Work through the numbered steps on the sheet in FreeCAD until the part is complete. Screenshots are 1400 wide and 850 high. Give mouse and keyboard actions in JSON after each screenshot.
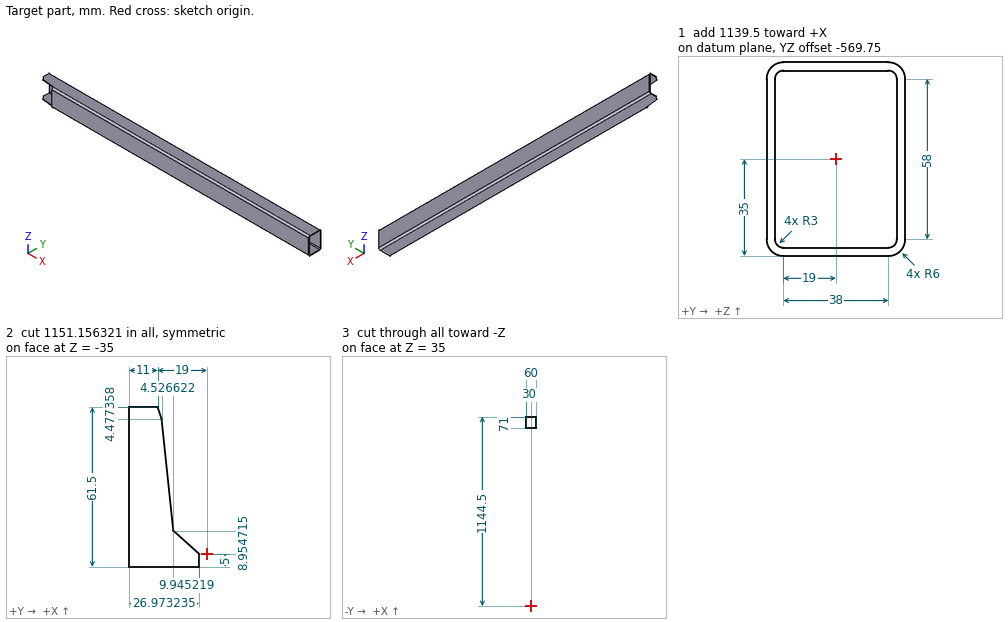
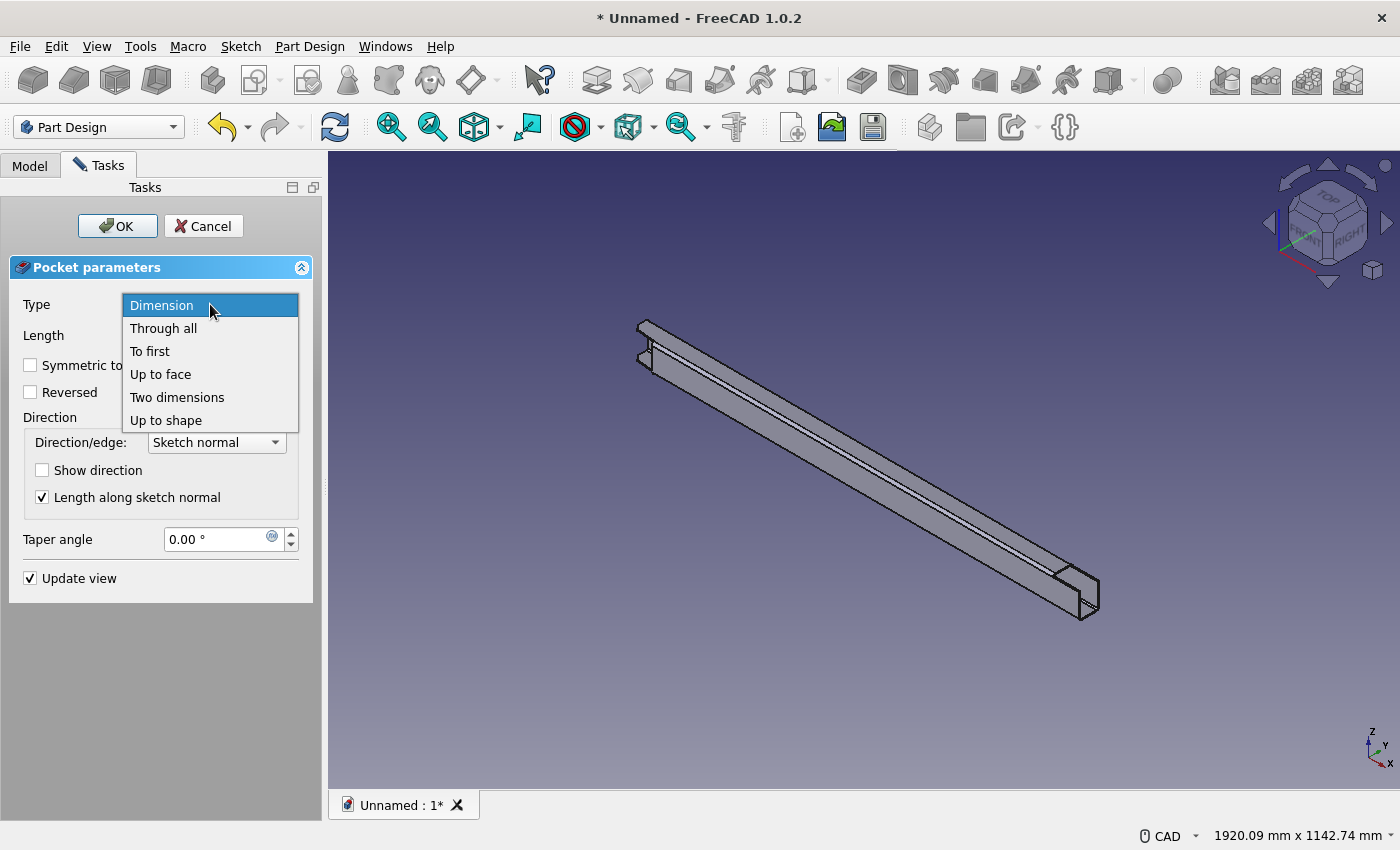
{"action": "left_click", "coordinate": [208, 328]}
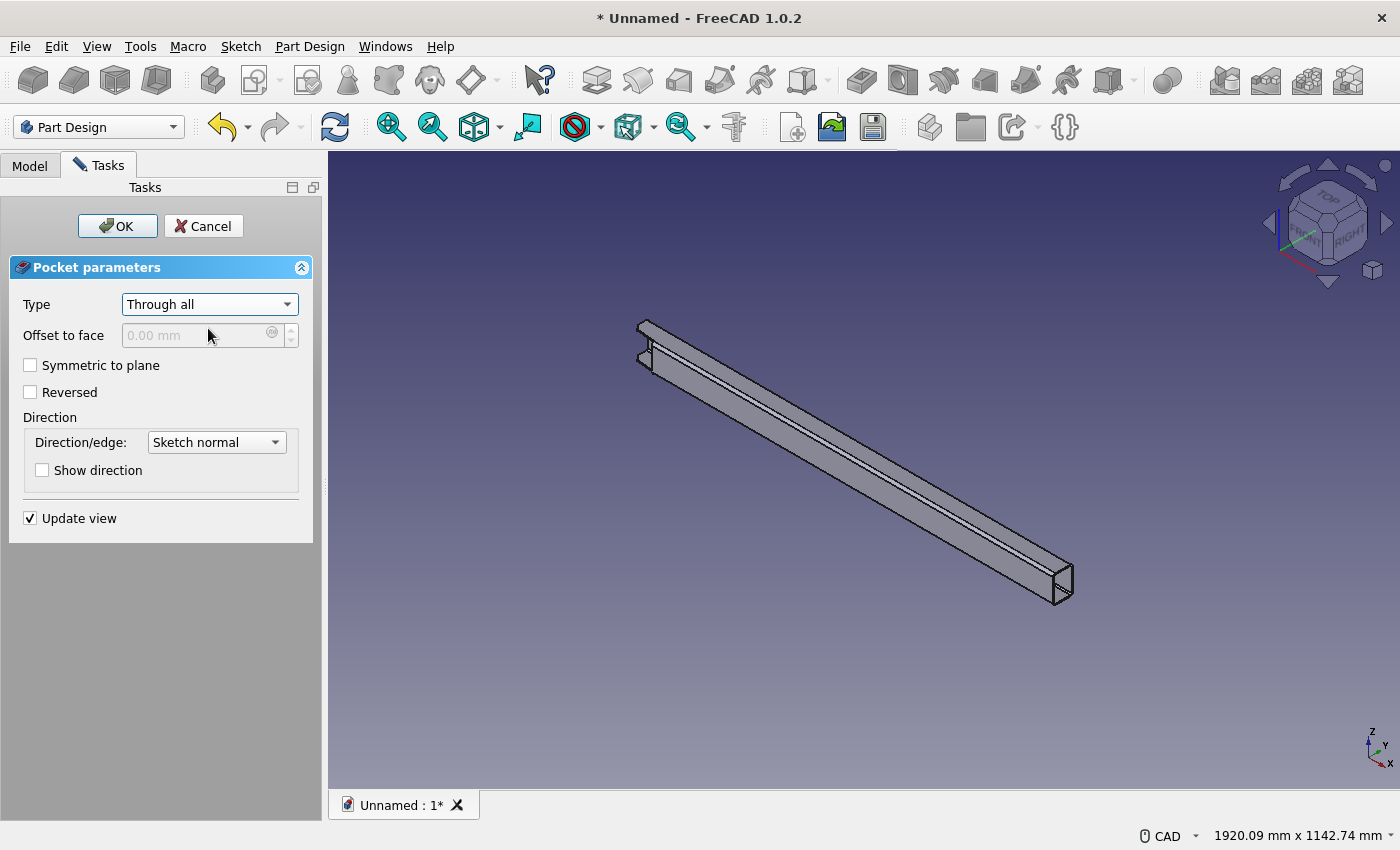
{"action": "left_click", "coordinate": [118, 226]}